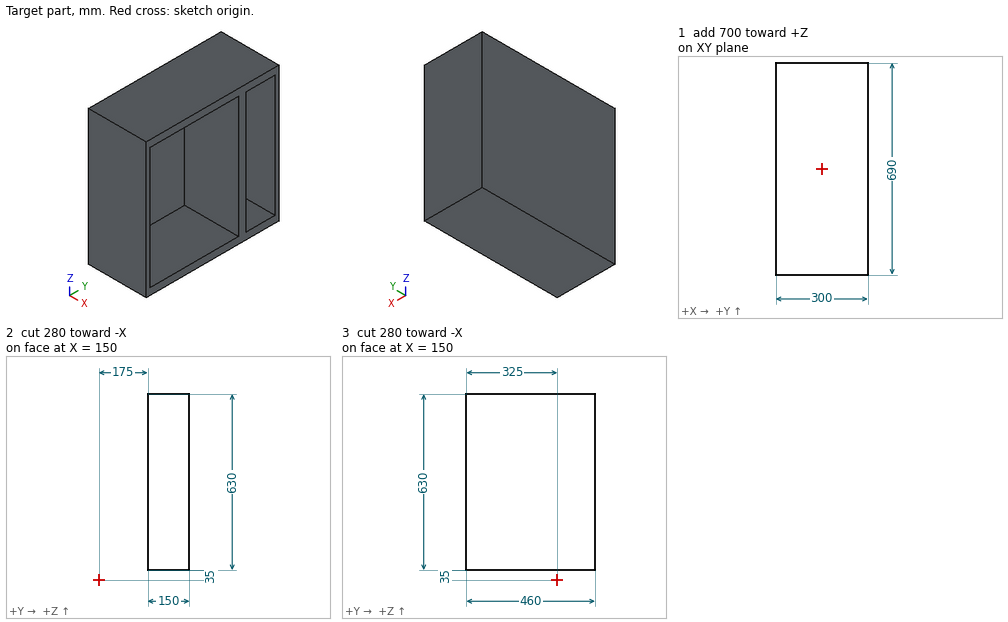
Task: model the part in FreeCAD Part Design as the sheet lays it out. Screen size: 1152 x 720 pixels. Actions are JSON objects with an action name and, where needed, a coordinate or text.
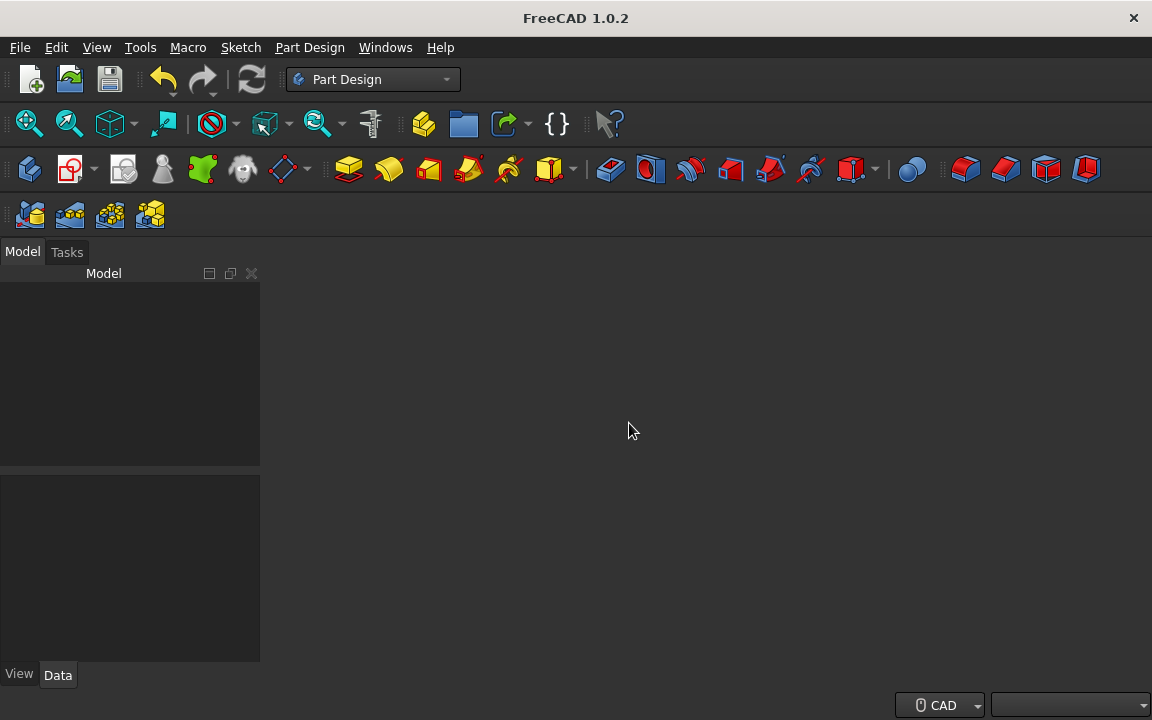
{"action": "key", "text": "ctrl+n"}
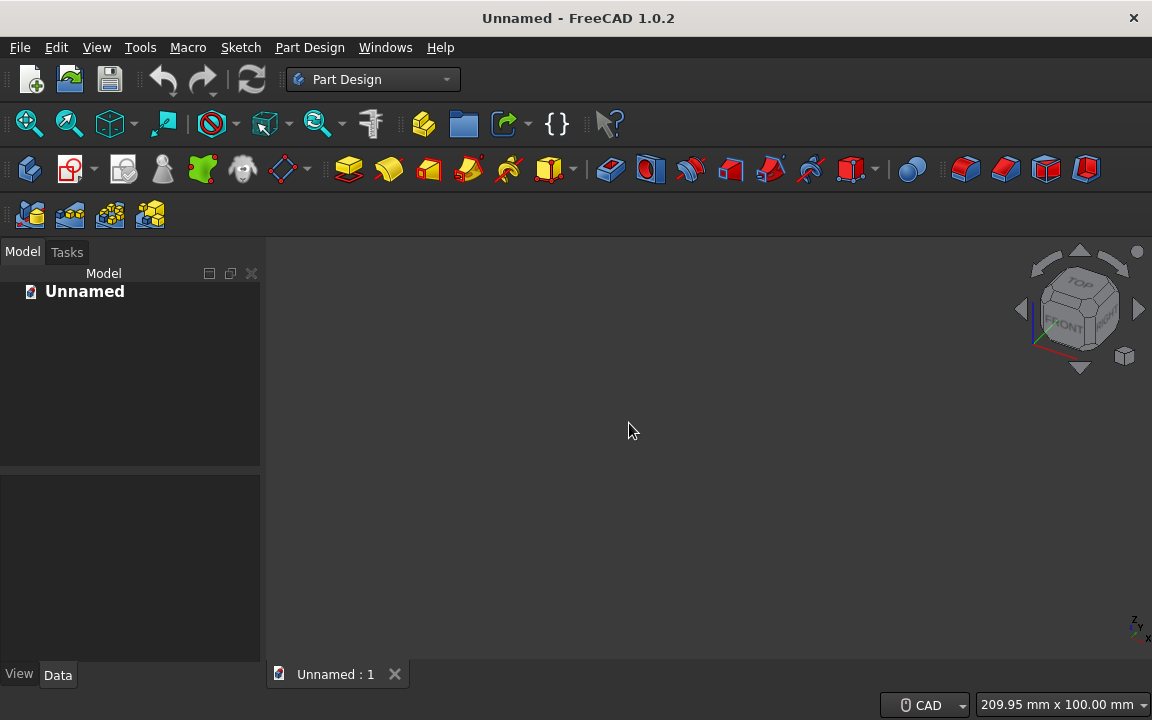
{"action": "left_click", "coordinate": [70, 170]}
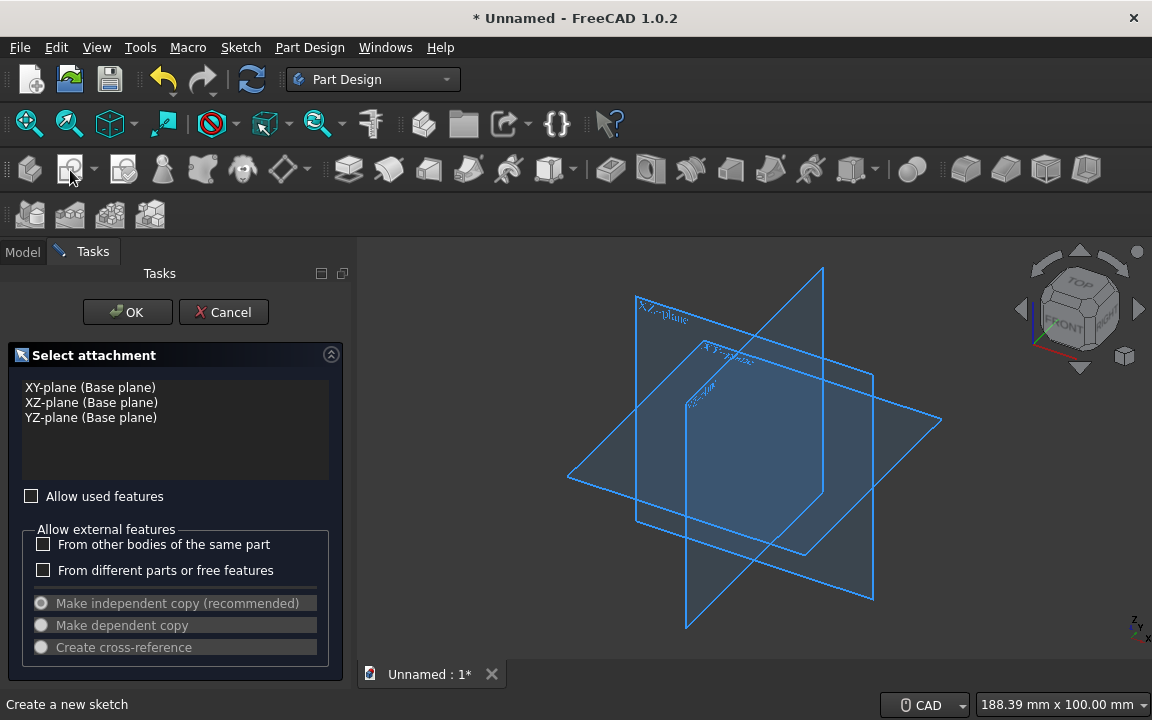
{"action": "left_click", "coordinate": [82, 388]}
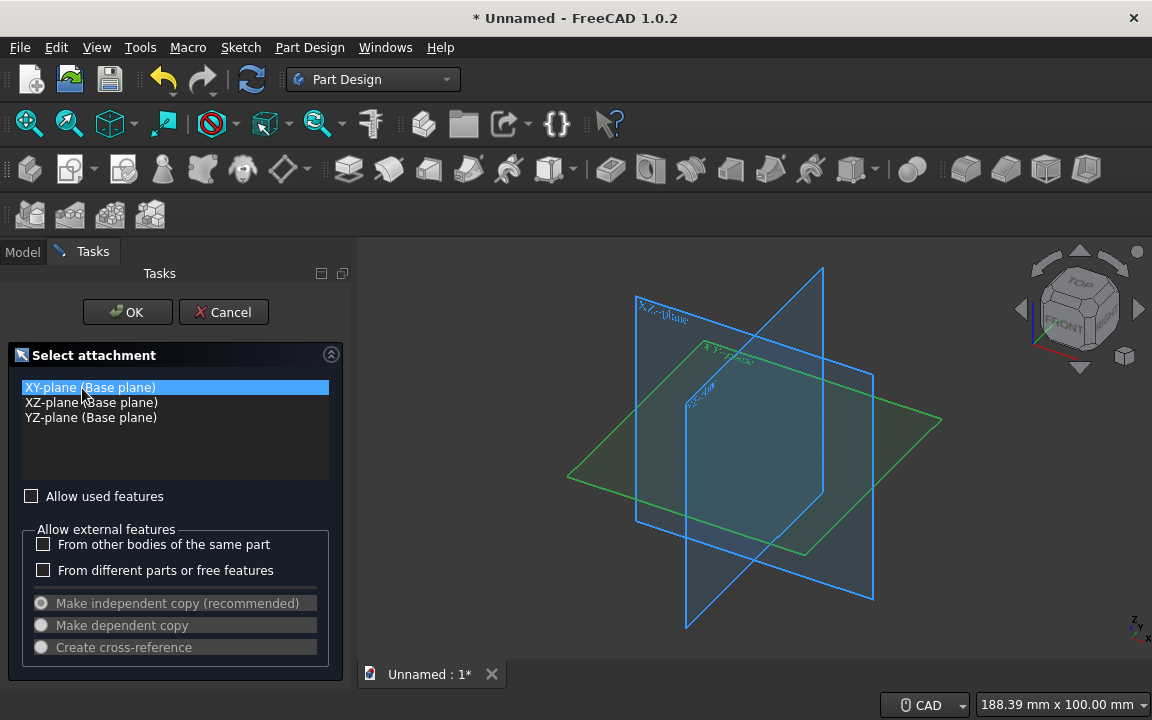
{"action": "left_click", "coordinate": [128, 312]}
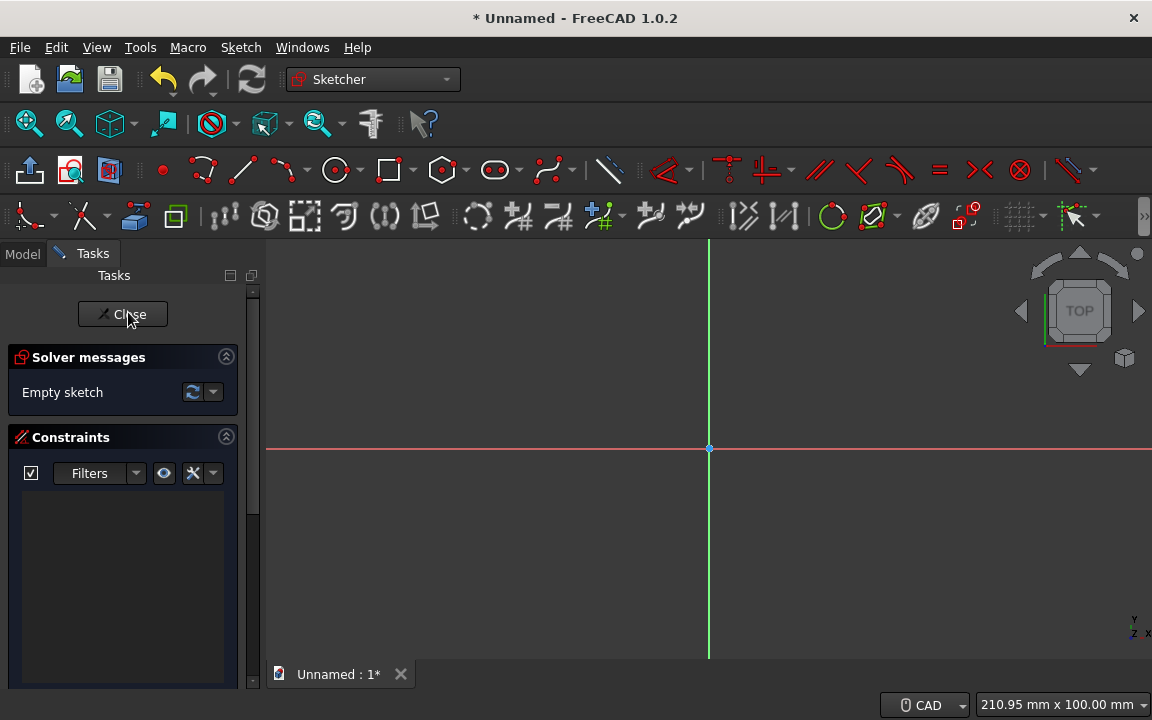
{"action": "scroll", "coordinate": [634, 449], "scroll_direction": "down", "scroll_amount": 12}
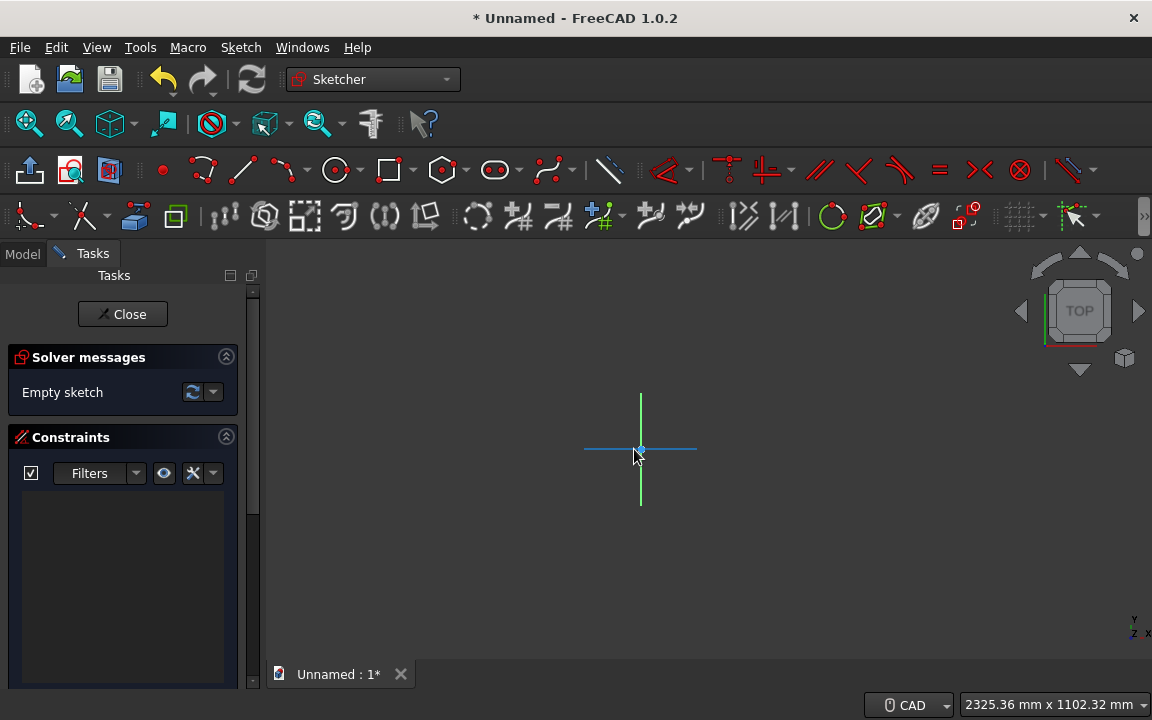
{"action": "key", "text": "g v"}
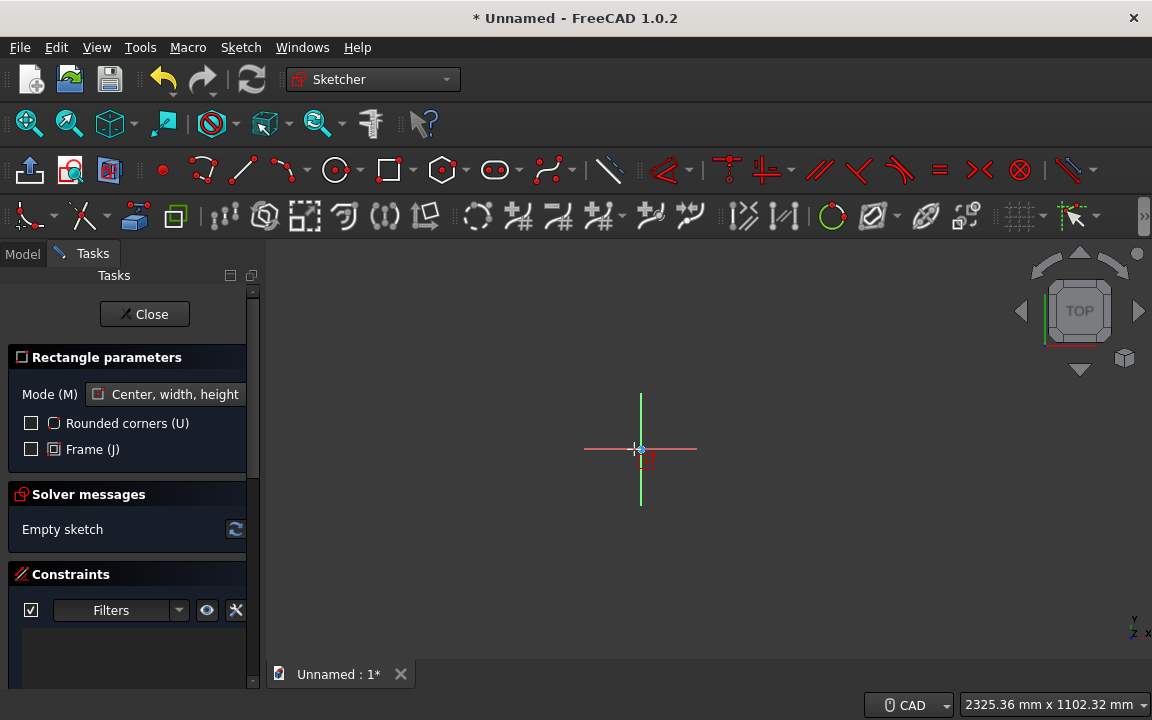
{"action": "left_click", "coordinate": [641, 449]}
{"action": "left_click", "coordinate": [698, 318]}
{"action": "key", "text": "Escape"}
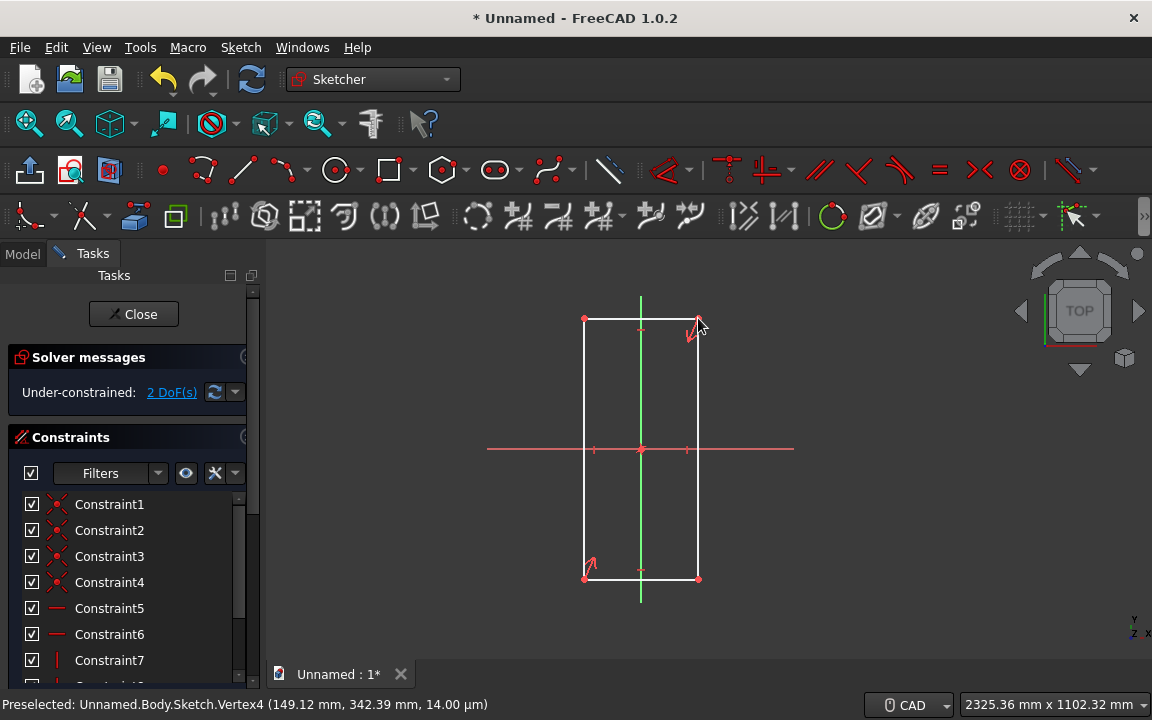
{"action": "left_click", "coordinate": [618, 580]}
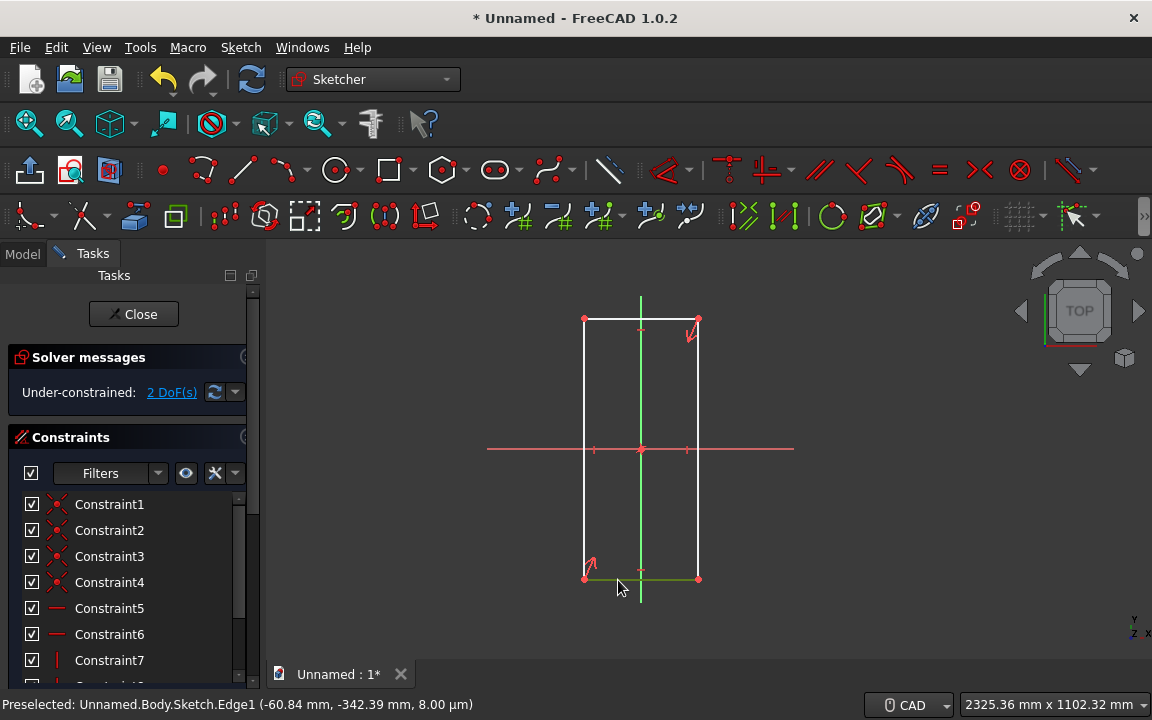
{"action": "key", "text": "l"}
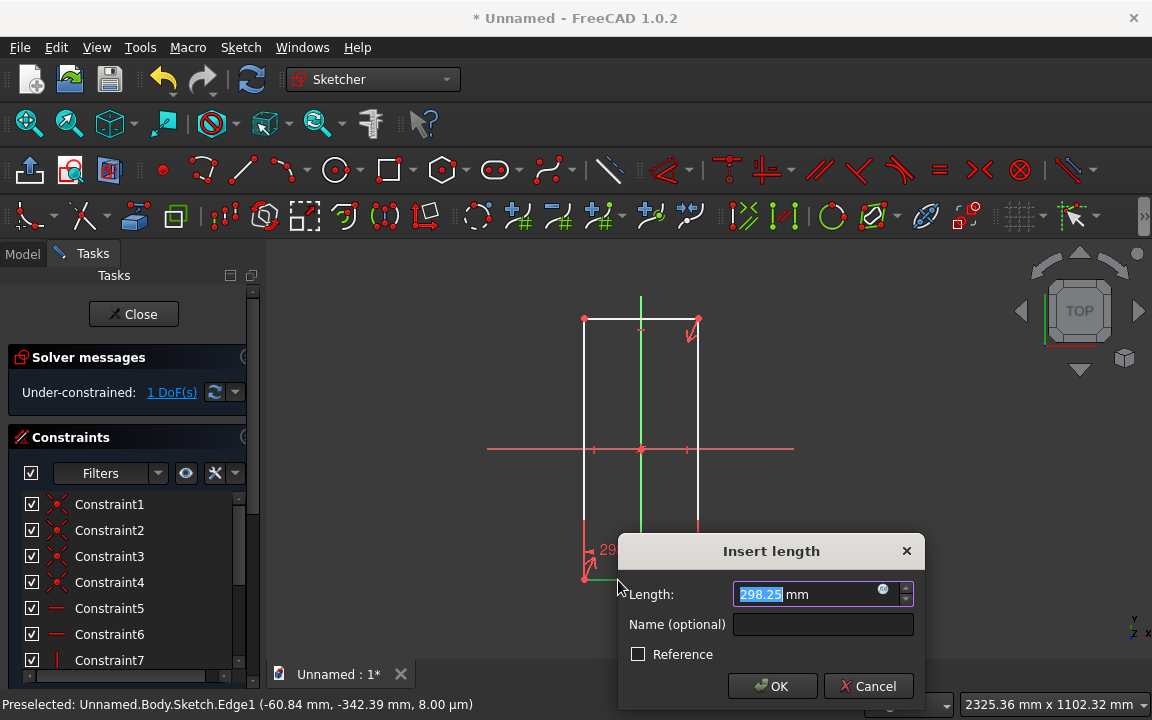
{"action": "type", "text": "300"}
{"action": "key", "text": "Return"}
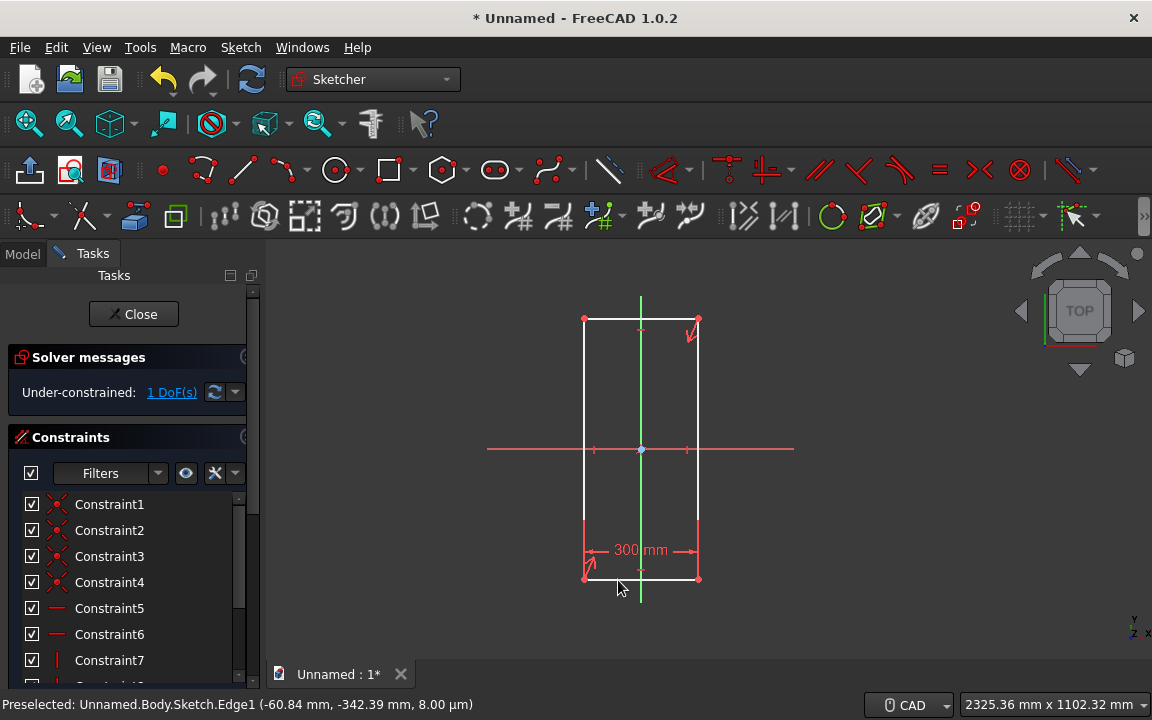
{"action": "left_click", "coordinate": [698, 502]}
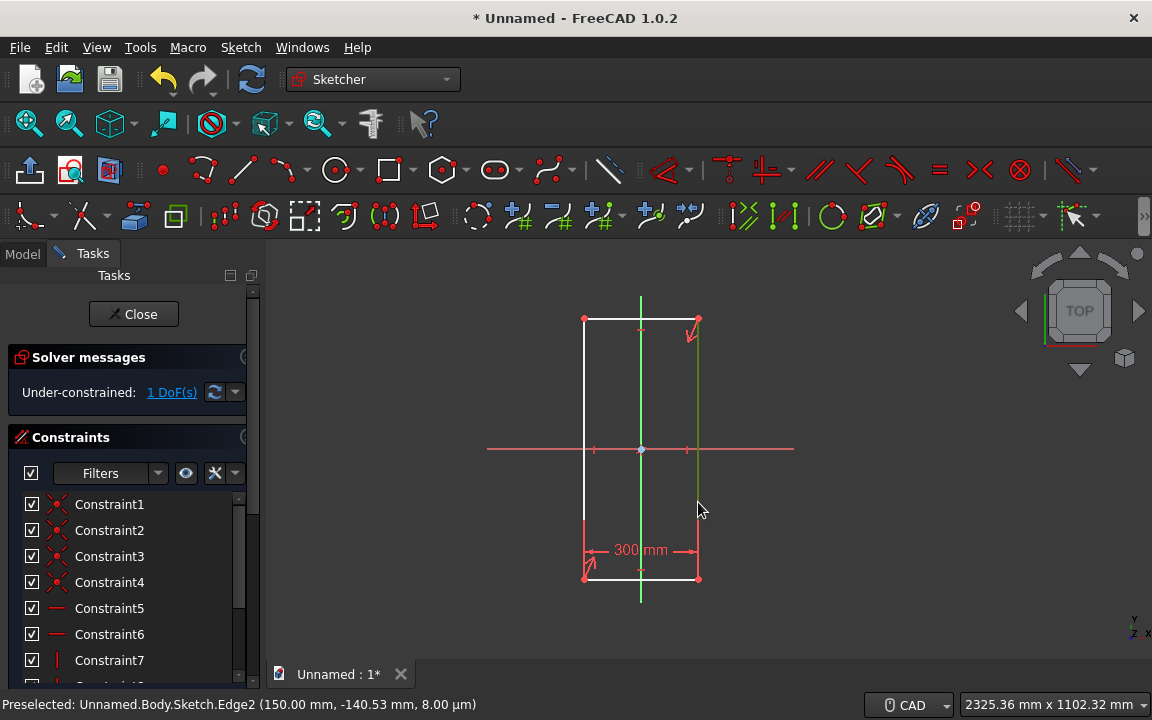
{"action": "left_click", "coordinate": [692, 170]}